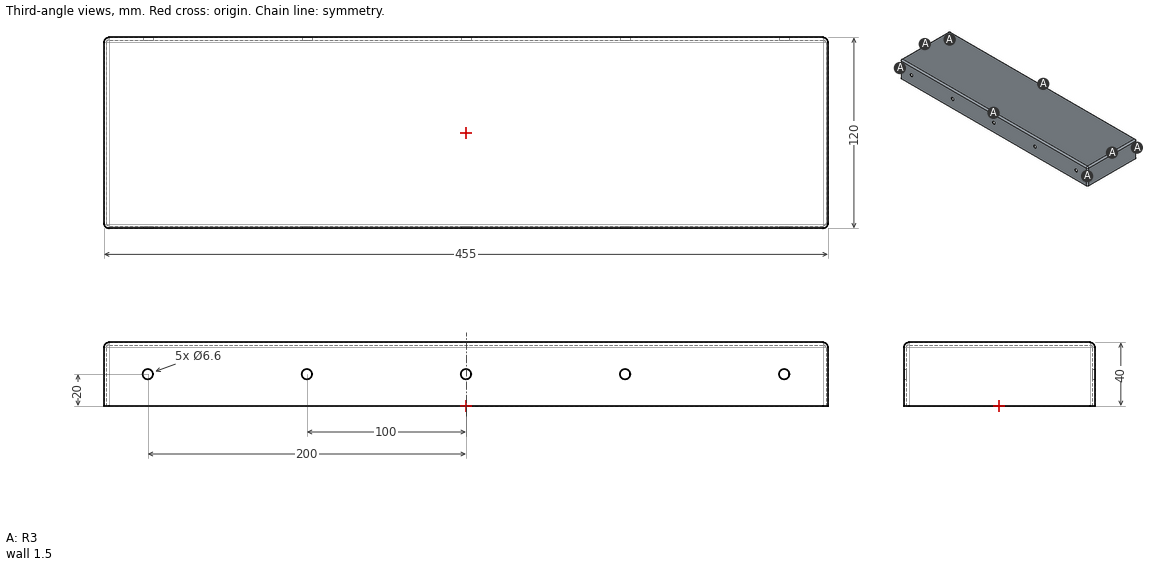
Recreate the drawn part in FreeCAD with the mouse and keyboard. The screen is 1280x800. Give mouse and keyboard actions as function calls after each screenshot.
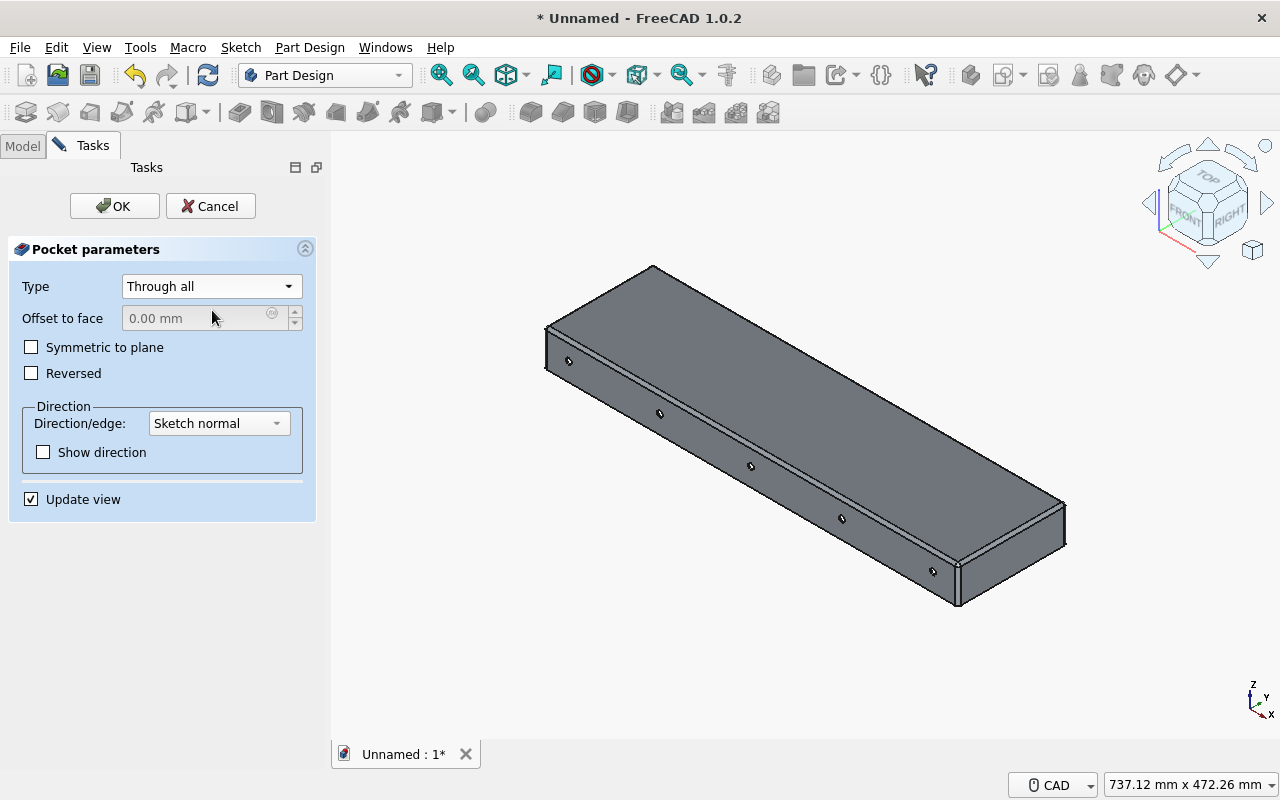
click(115, 206)